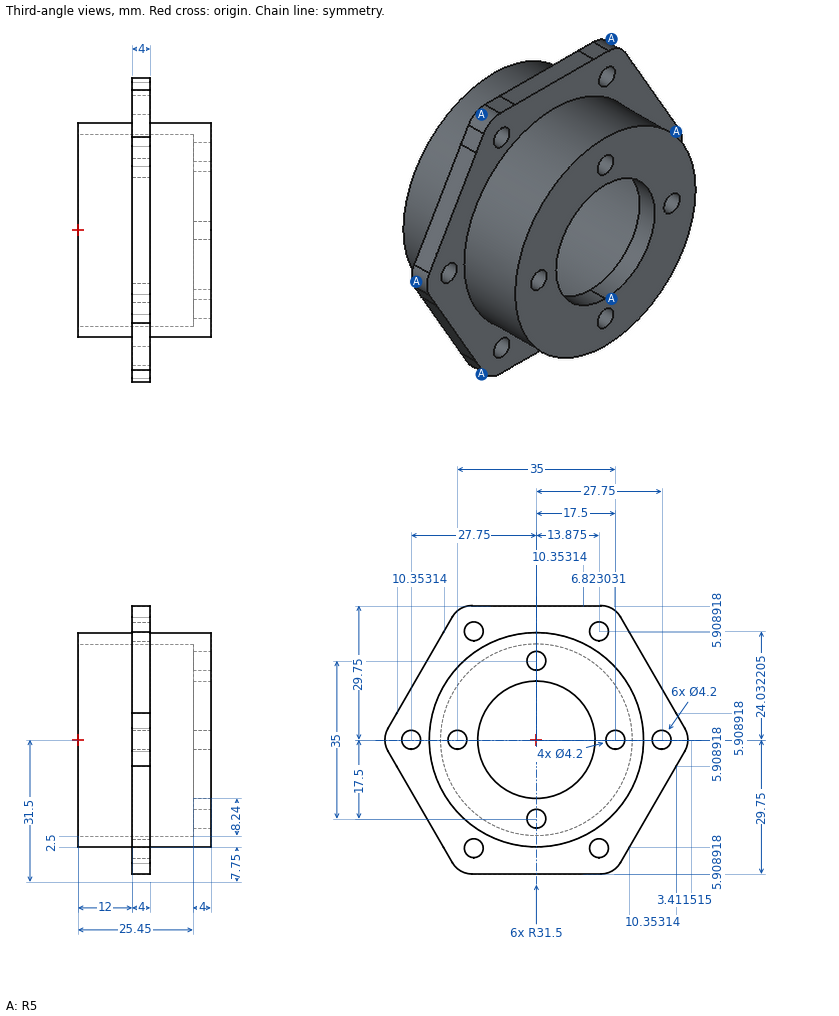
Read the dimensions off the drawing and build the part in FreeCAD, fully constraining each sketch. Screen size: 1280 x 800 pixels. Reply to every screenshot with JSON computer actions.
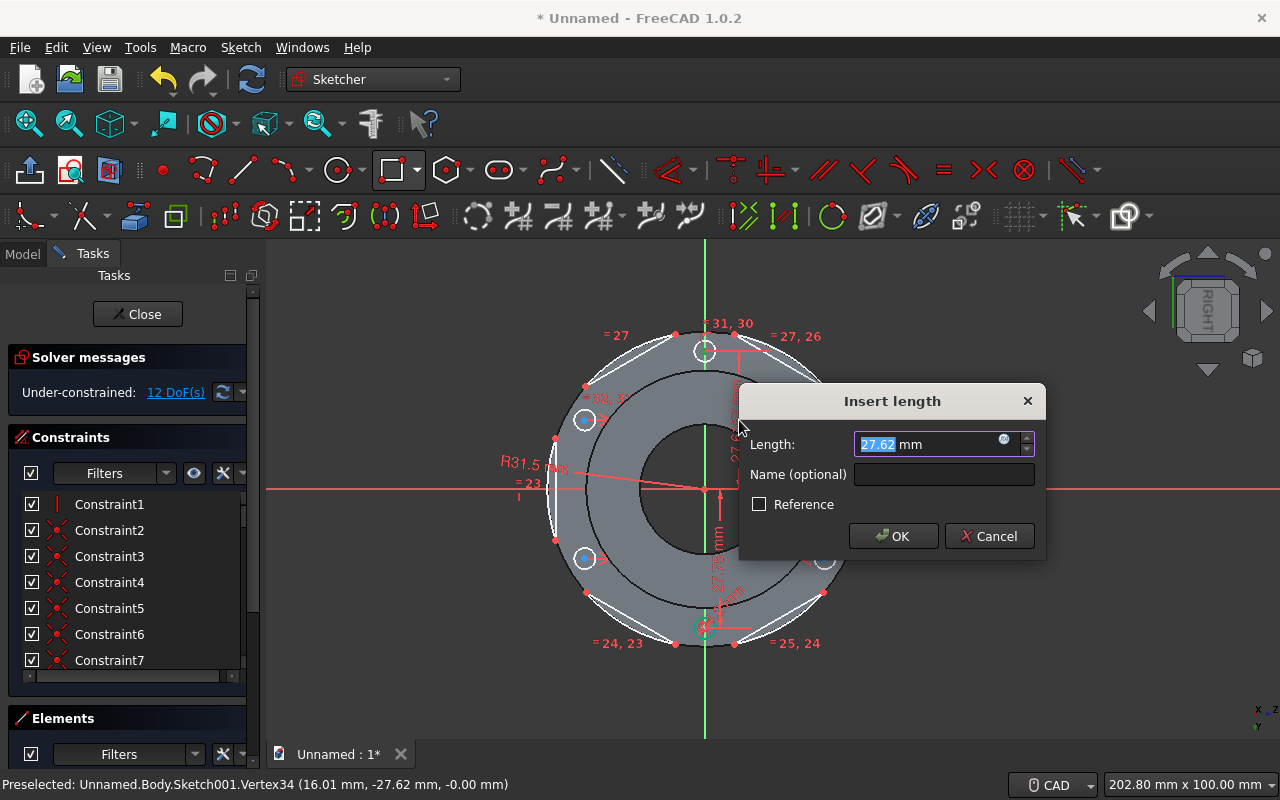
{"action": "type", "text": "27.75"}
{"action": "key", "text": "Return"}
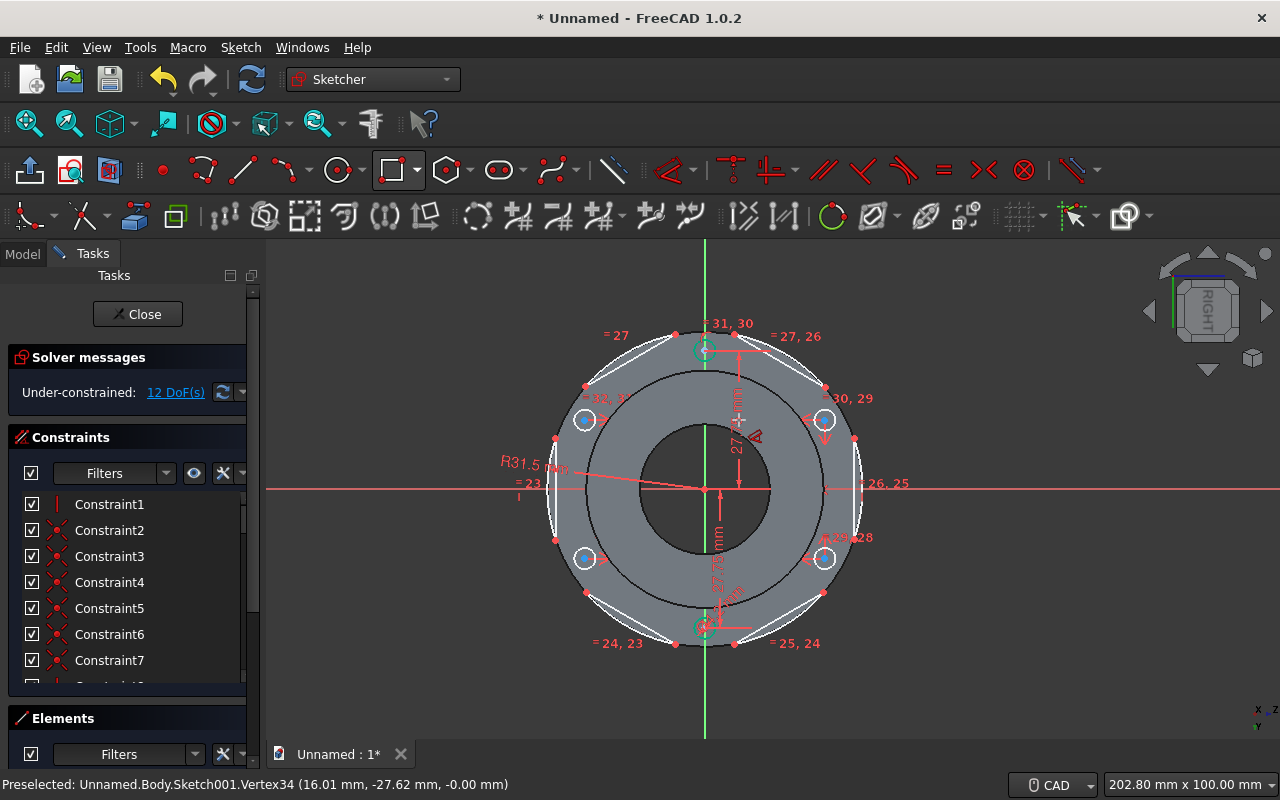
{"action": "left_click", "coordinate": [556, 540]}
{"action": "left_click", "coordinate": [630, 574]}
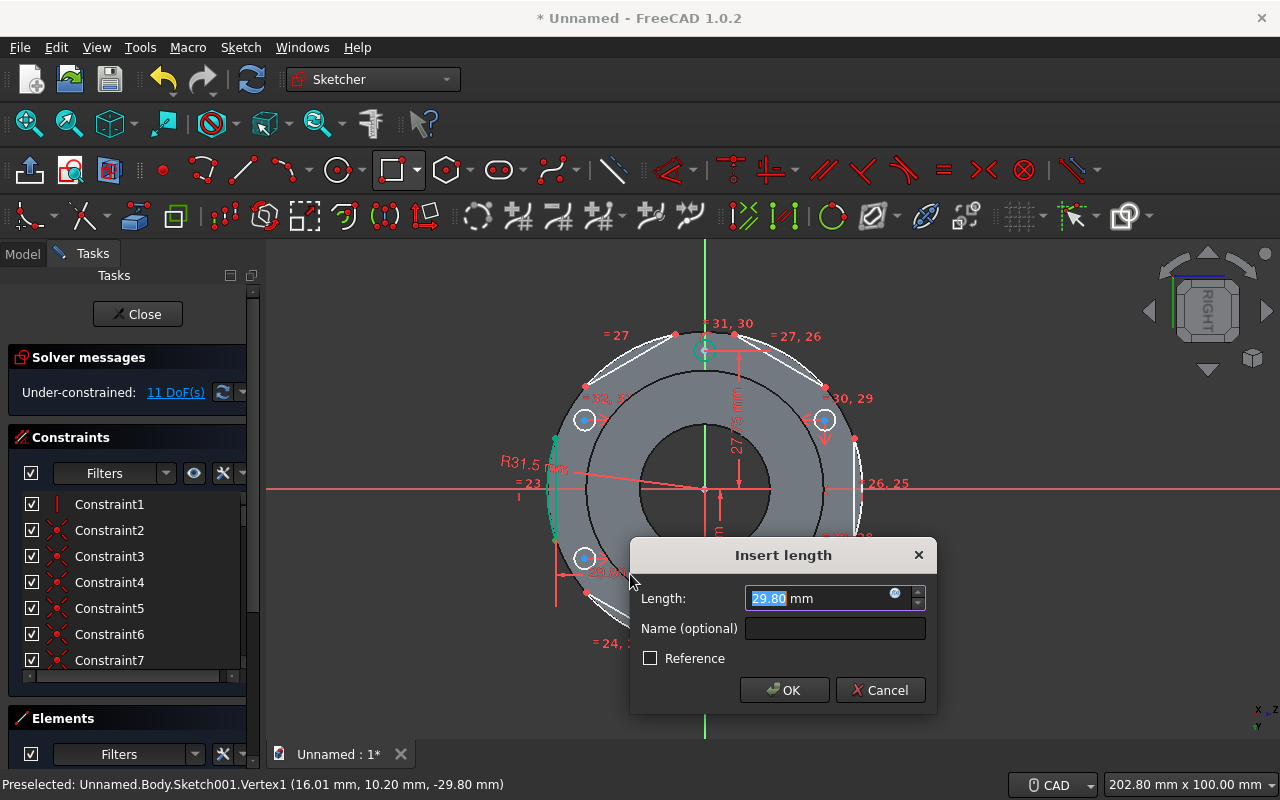
{"action": "type", "text": "29.75"}
{"action": "key", "text": "Return"}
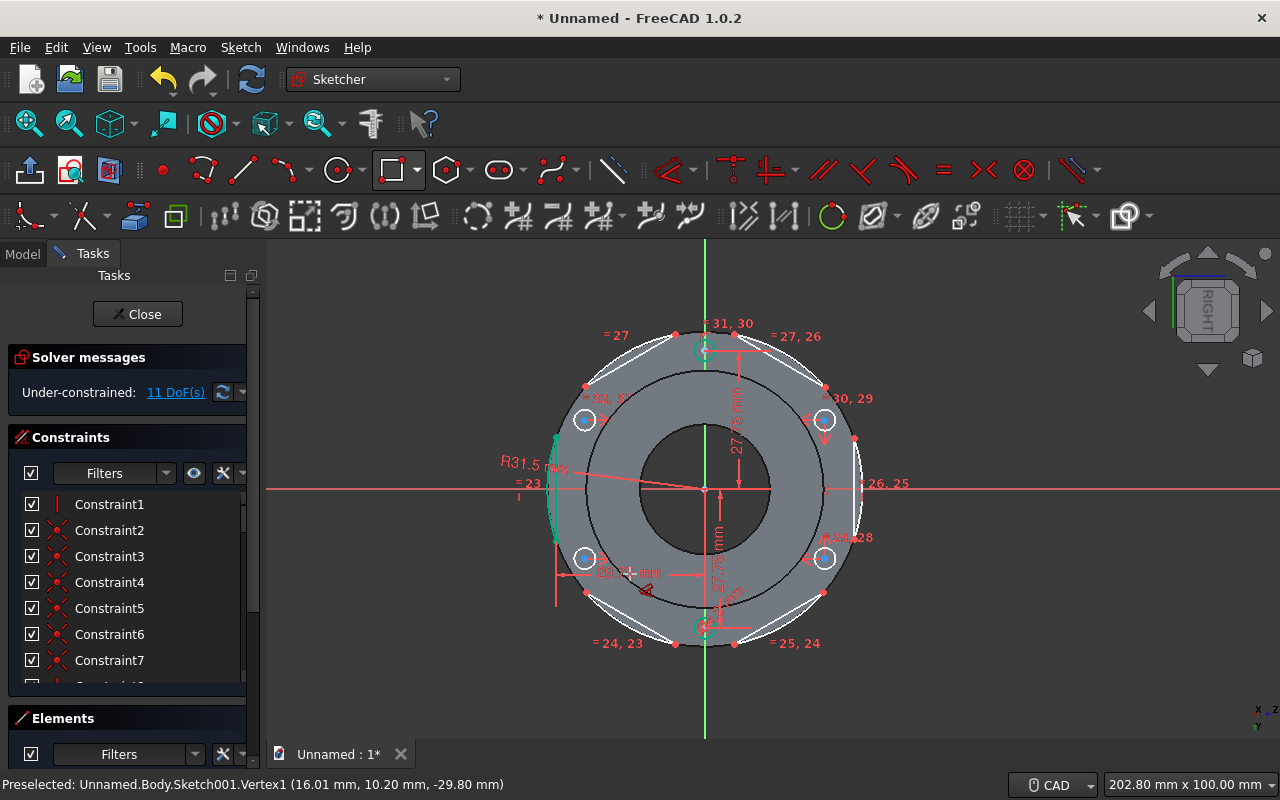
{"action": "left_click", "coordinate": [854, 439]}
{"action": "left_click", "coordinate": [779, 523]}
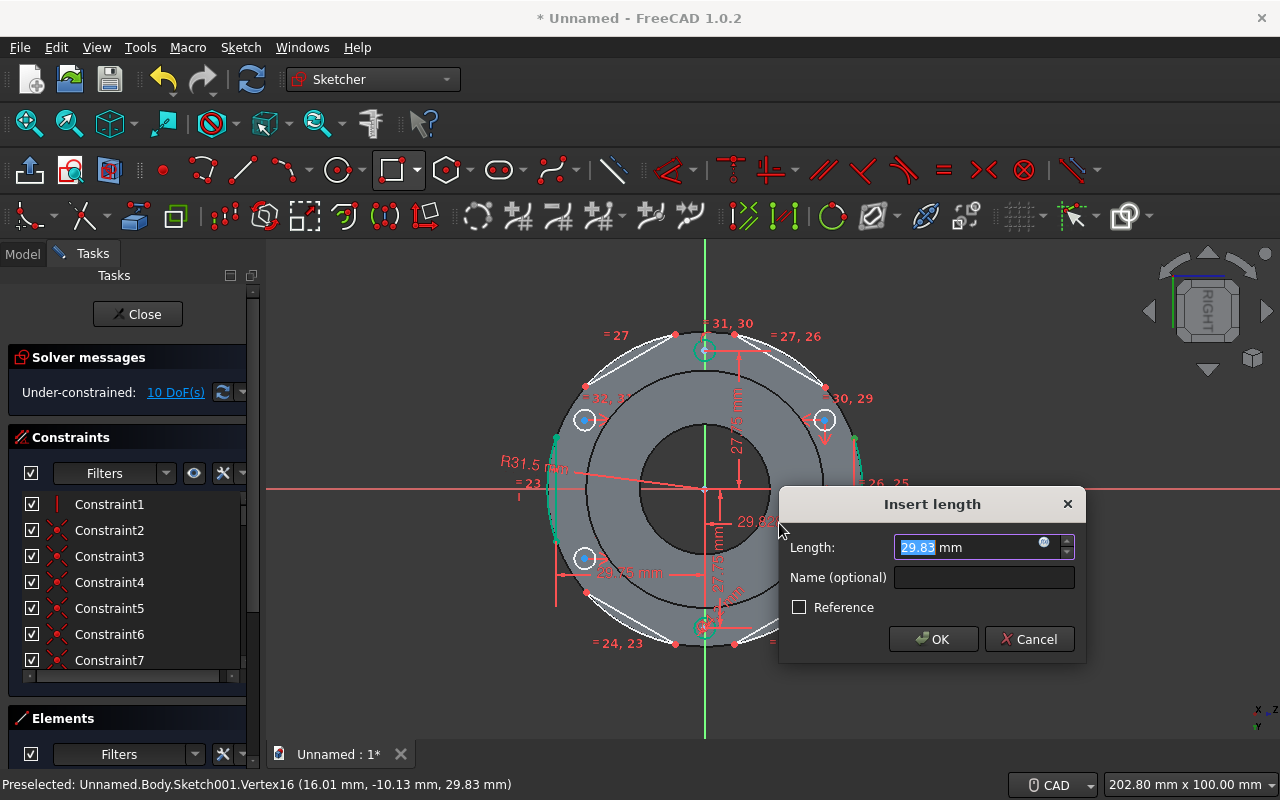
{"action": "type", "text": "29.75"}
{"action": "key", "text": "Return"}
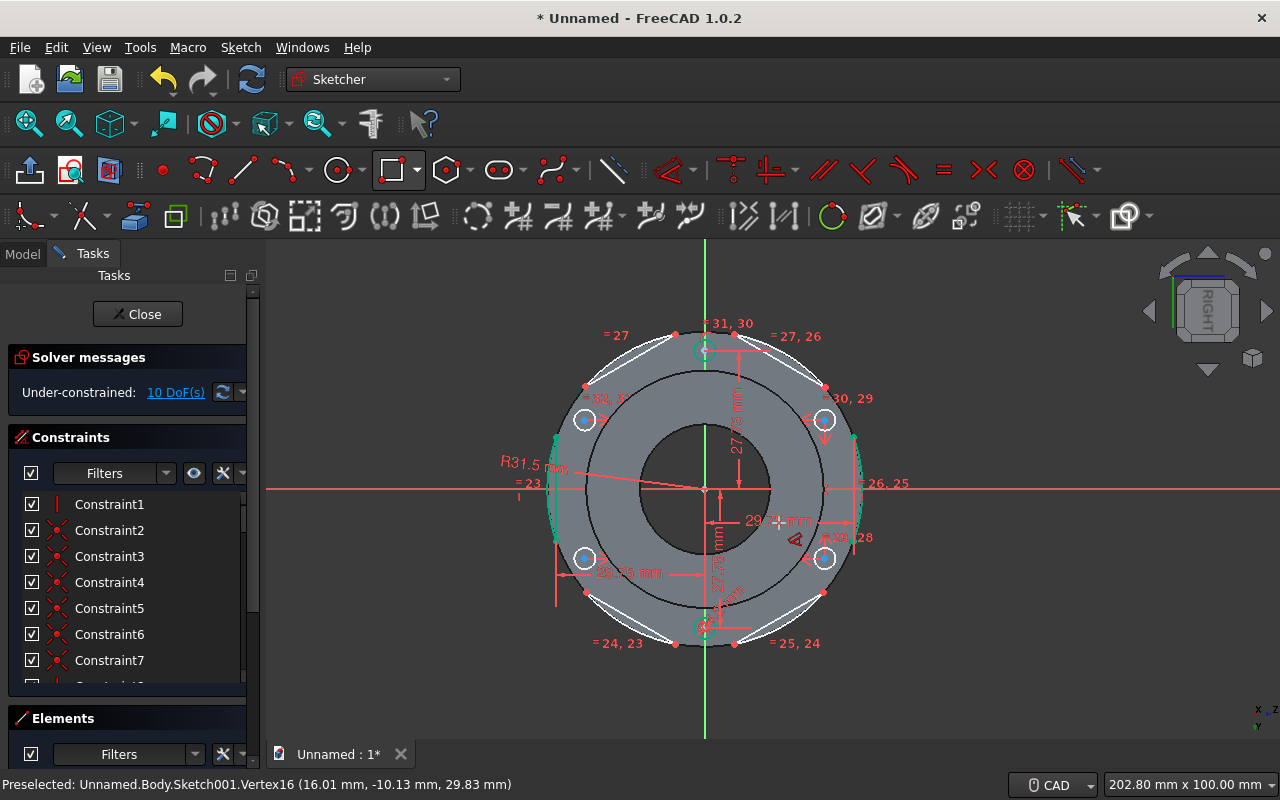
{"action": "left_click", "coordinate": [825, 559]}
{"action": "left_click", "coordinate": [671, 524]}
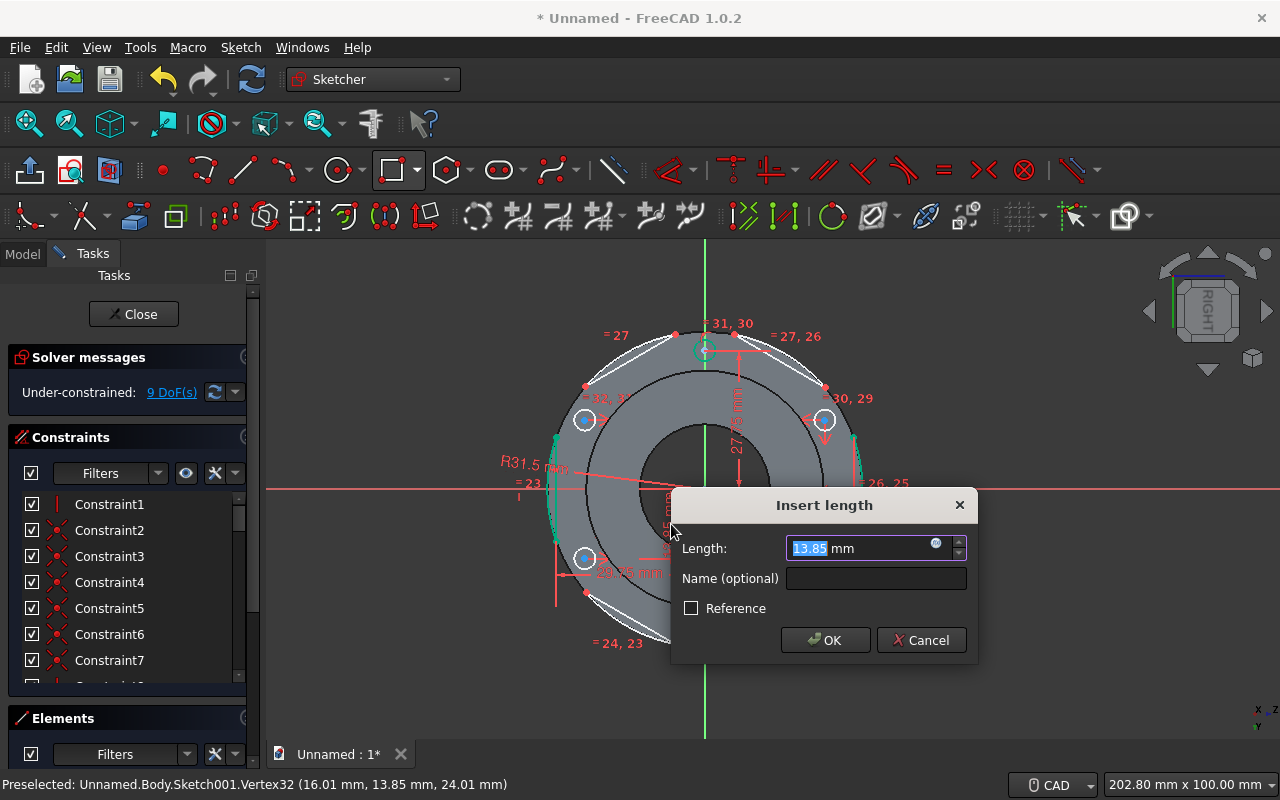
{"action": "type", "text": "13.875"}
{"action": "key", "text": "Return"}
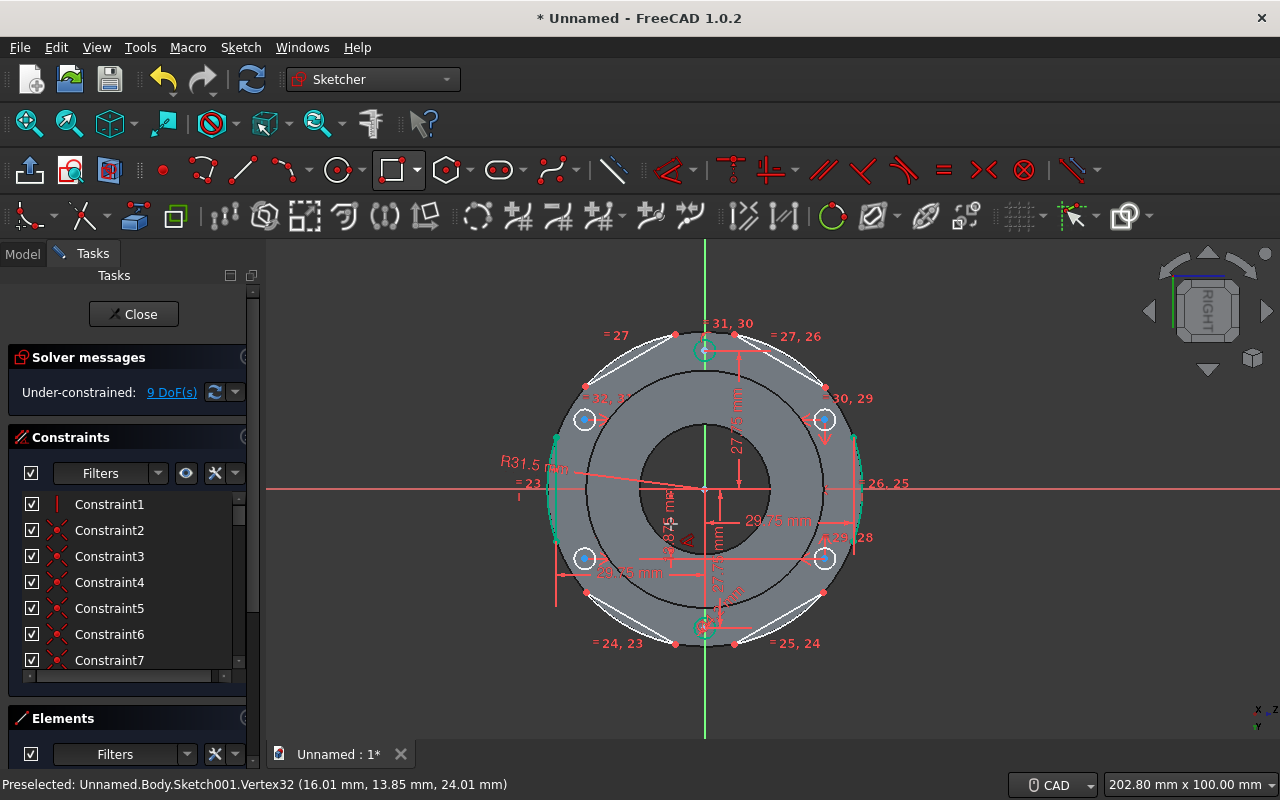
{"action": "scroll", "coordinate": [675, 644], "scroll_direction": "up", "scroll_amount": 2}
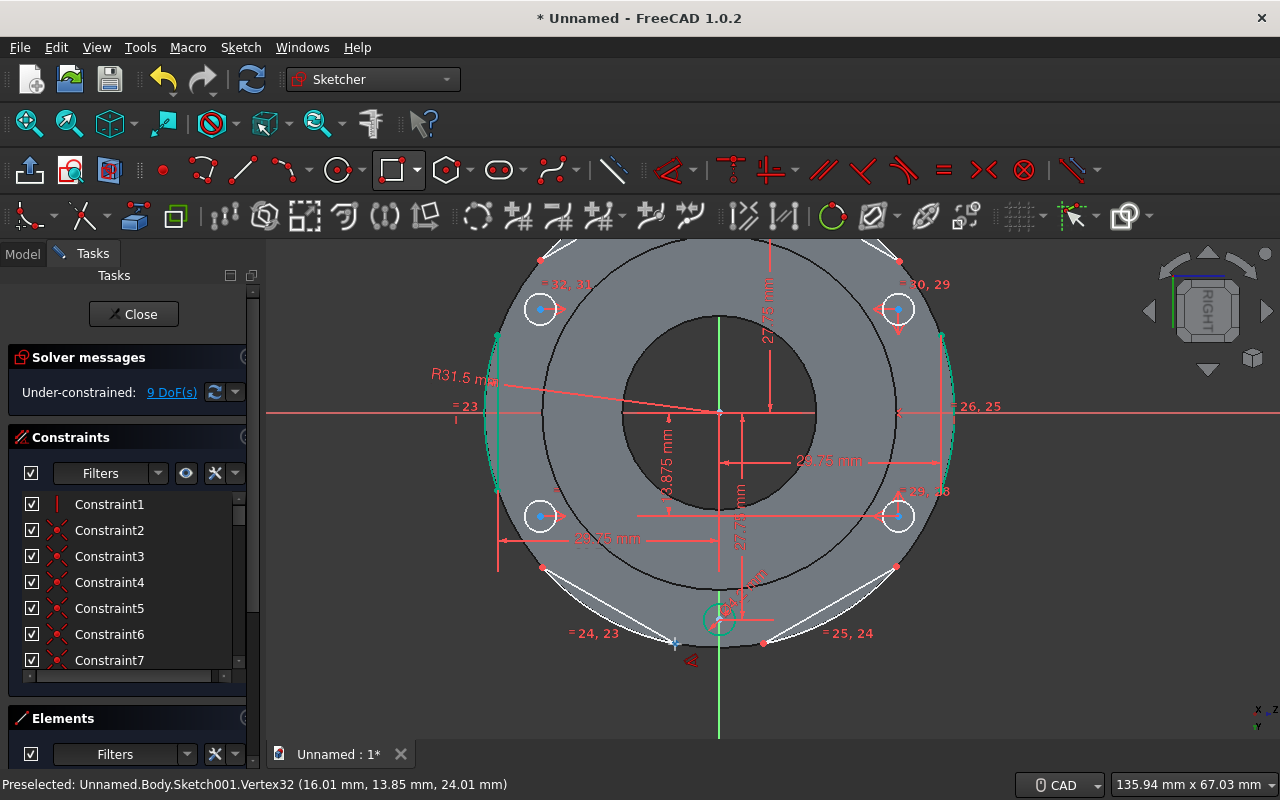
{"action": "left_click", "coordinate": [675, 644]}
{"action": "left_click", "coordinate": [697, 678]}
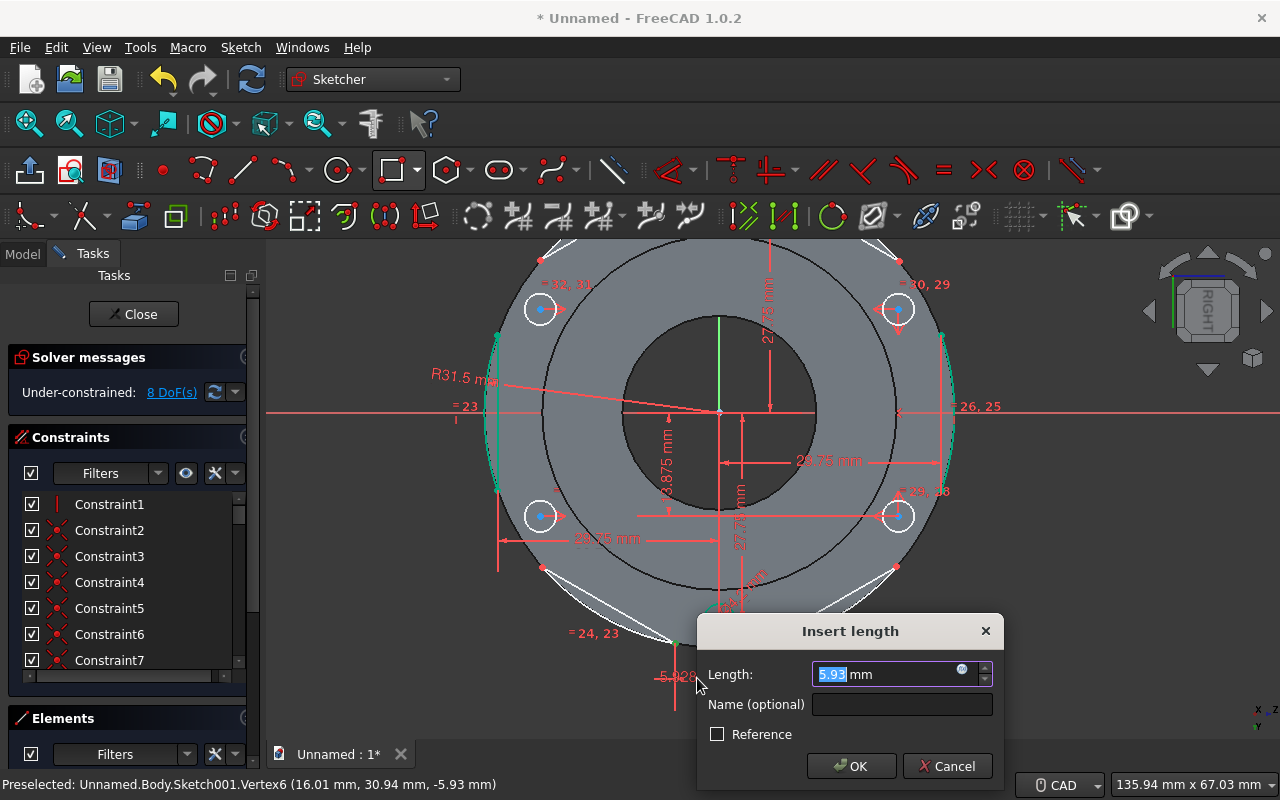
{"action": "type", "text": "5.908918"}
{"action": "key", "text": "Return"}